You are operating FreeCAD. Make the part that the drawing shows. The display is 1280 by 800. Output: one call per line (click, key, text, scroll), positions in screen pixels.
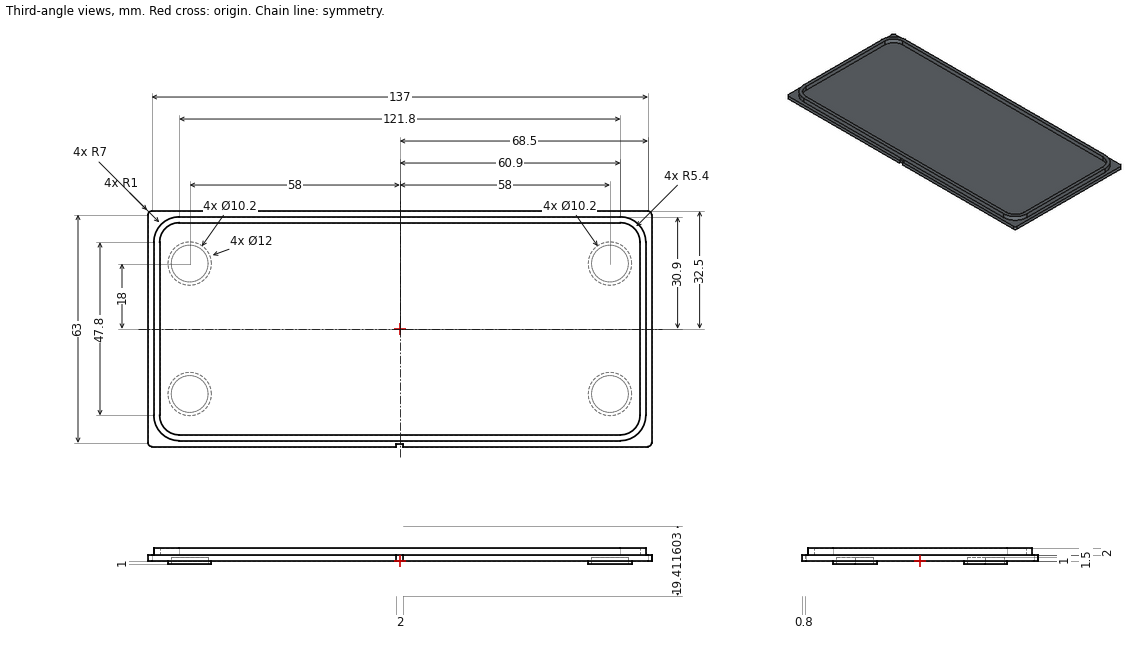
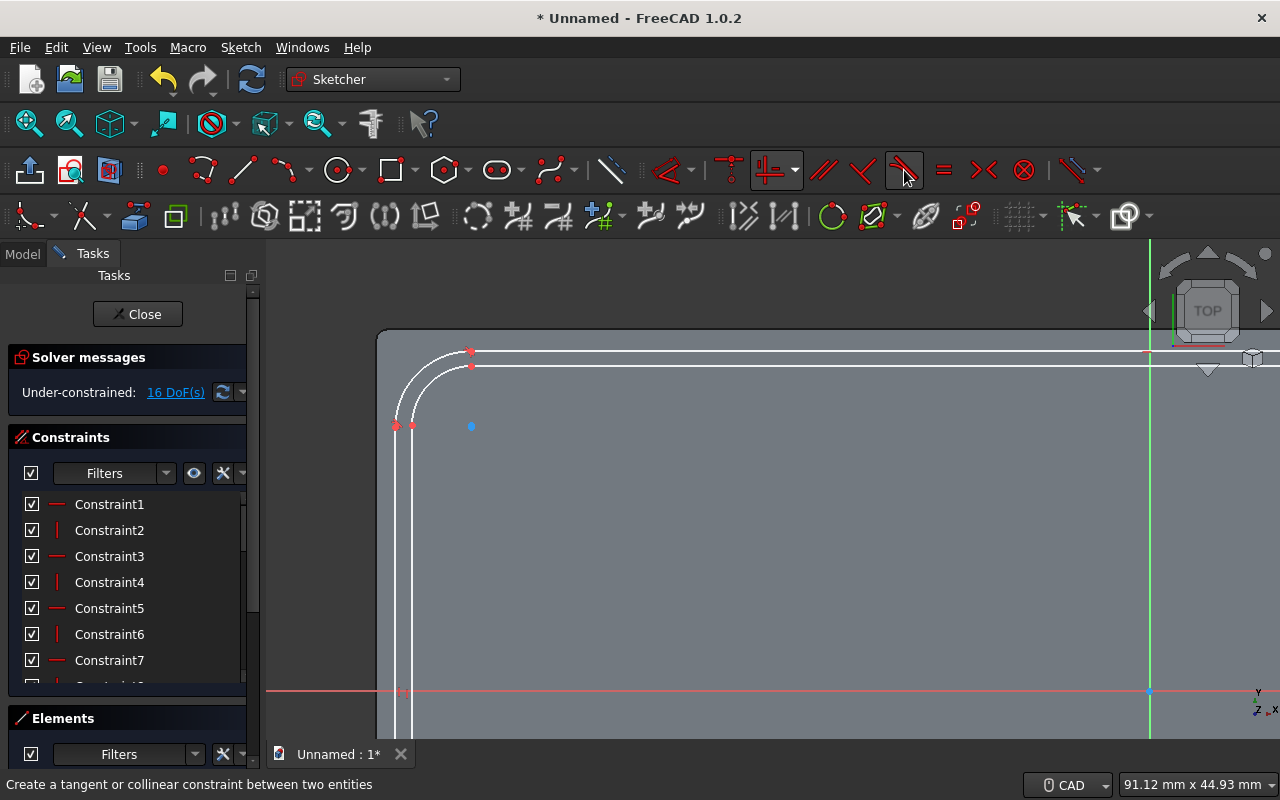
scroll(445, 371, down, 5)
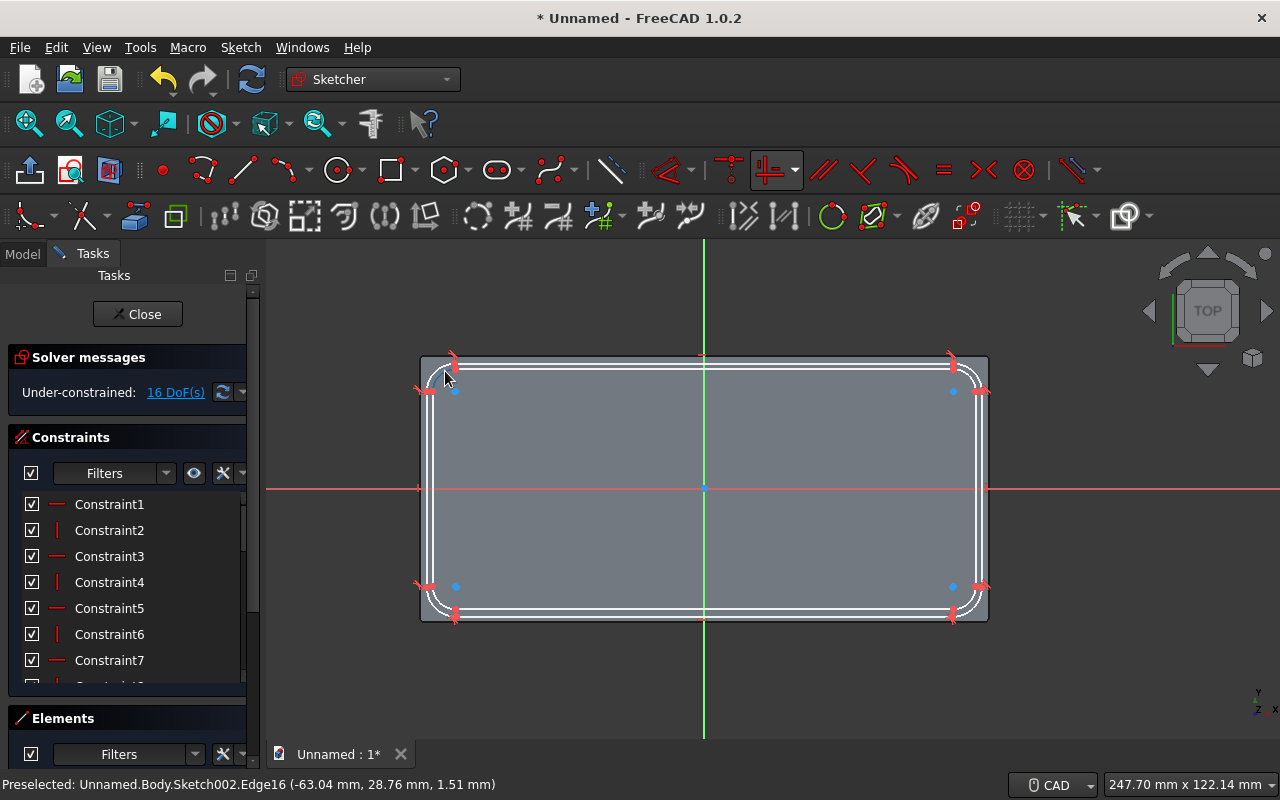
scroll(979, 379, up, 5)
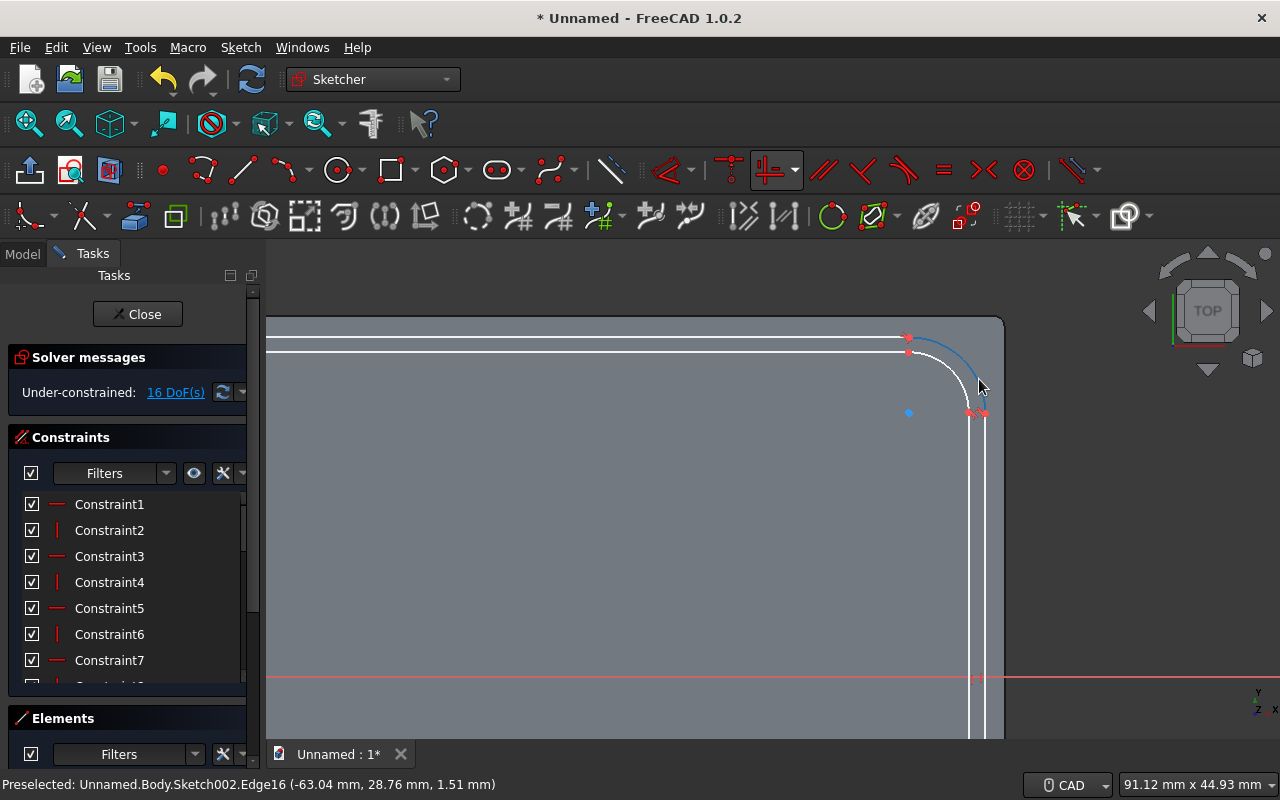
click(977, 379)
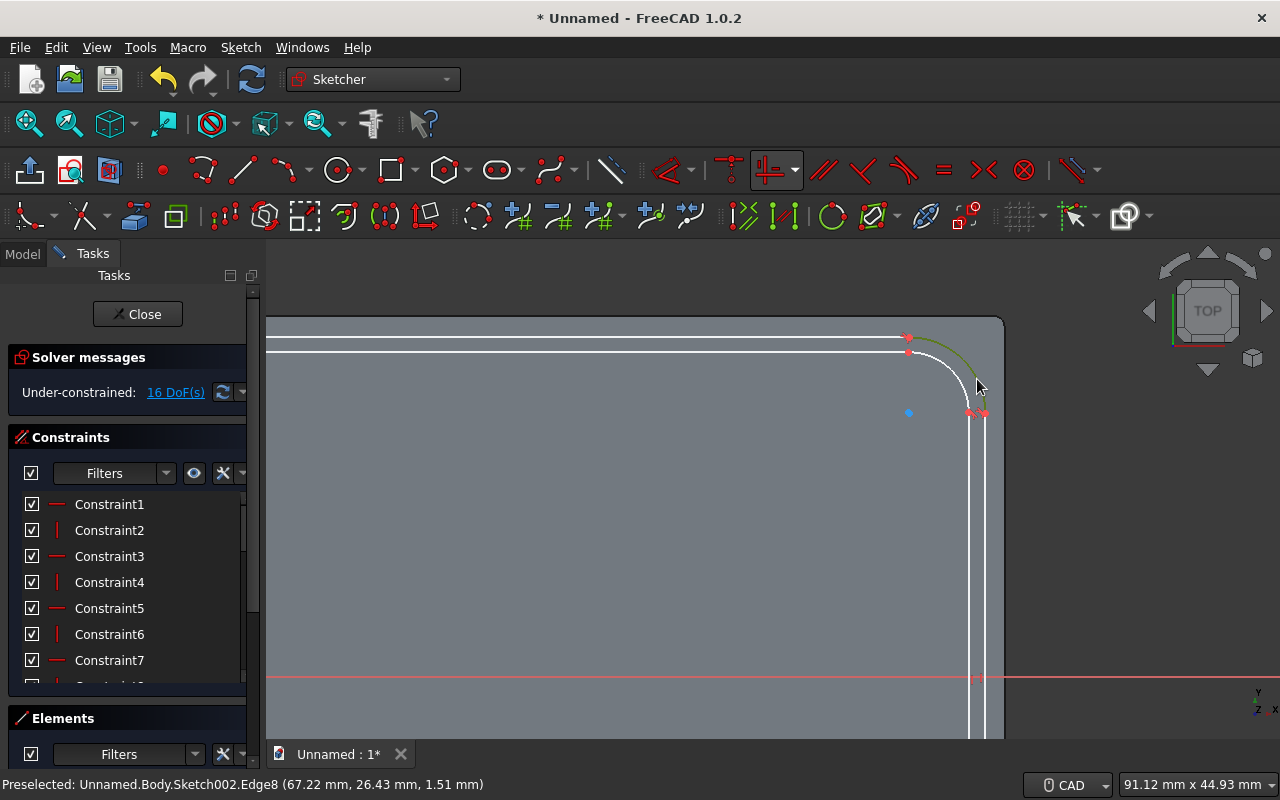
click(962, 385)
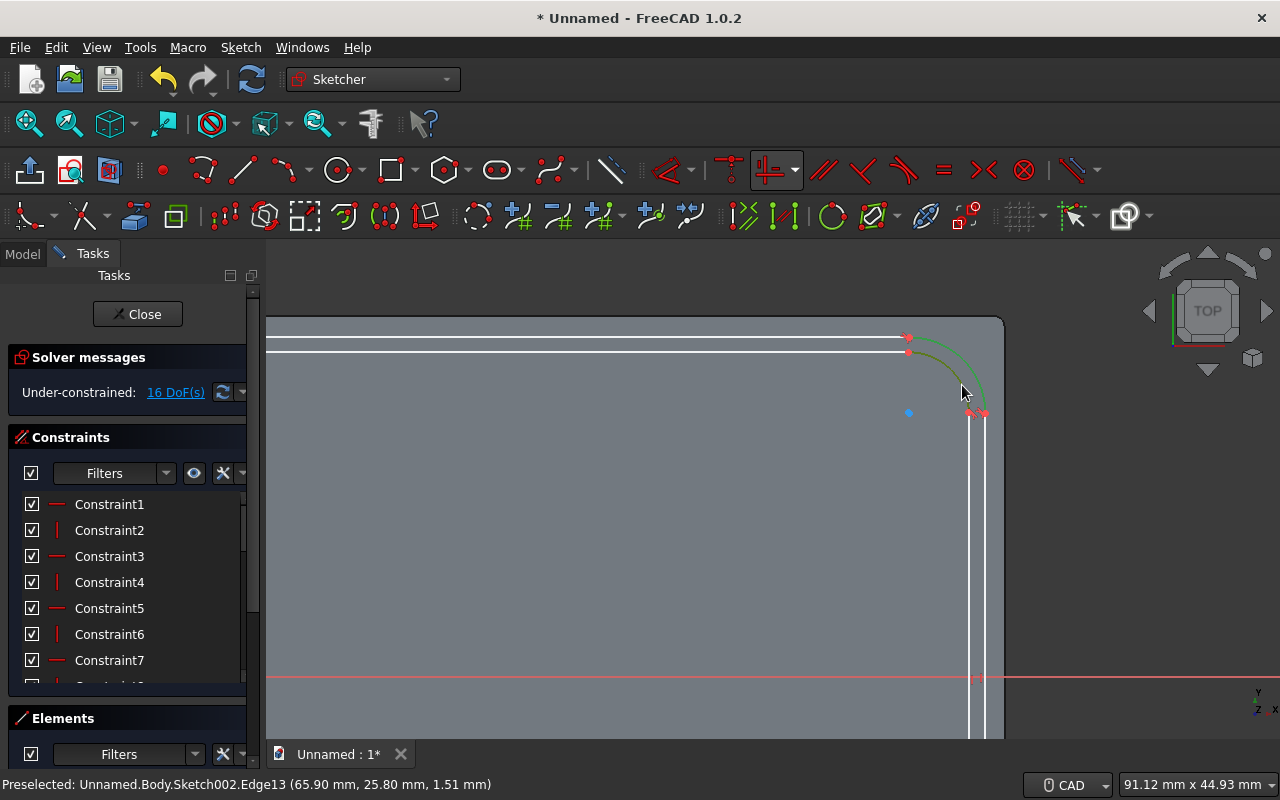
click(730, 170)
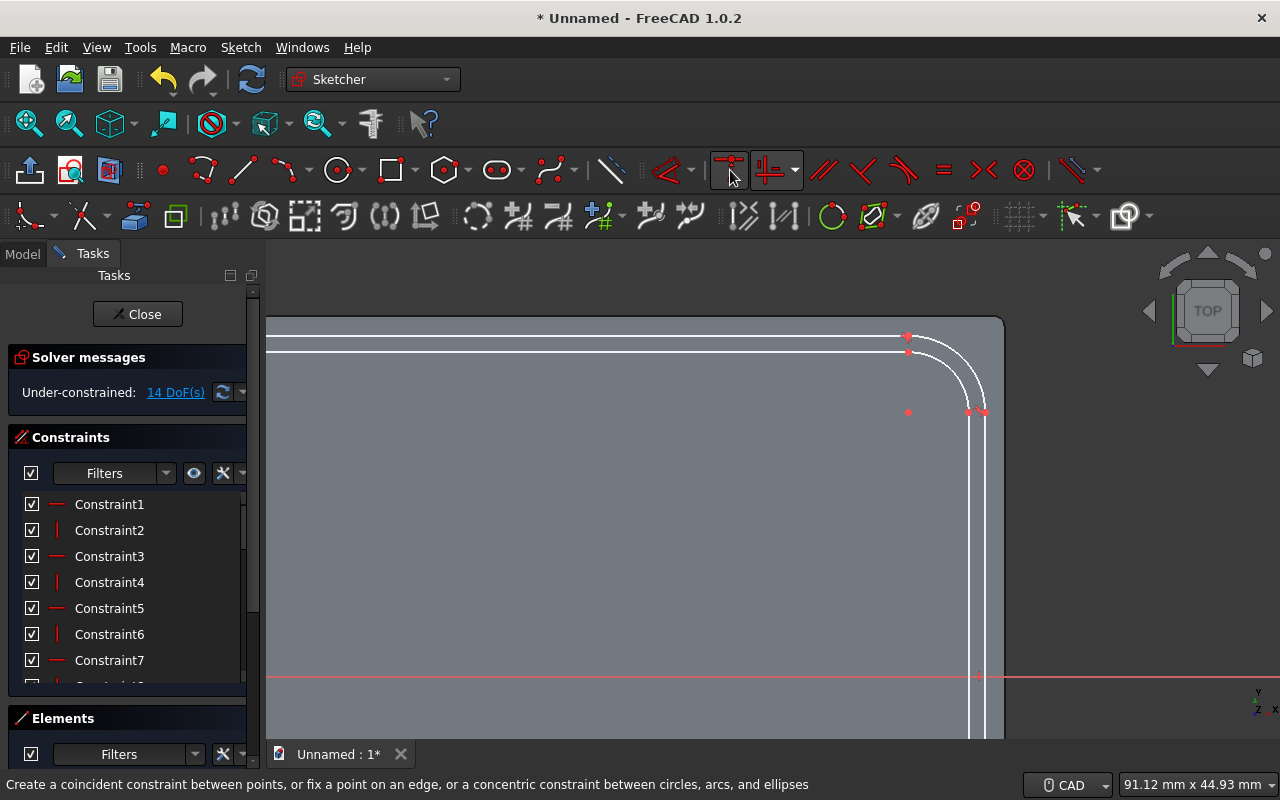
scroll(980, 379, down, 5)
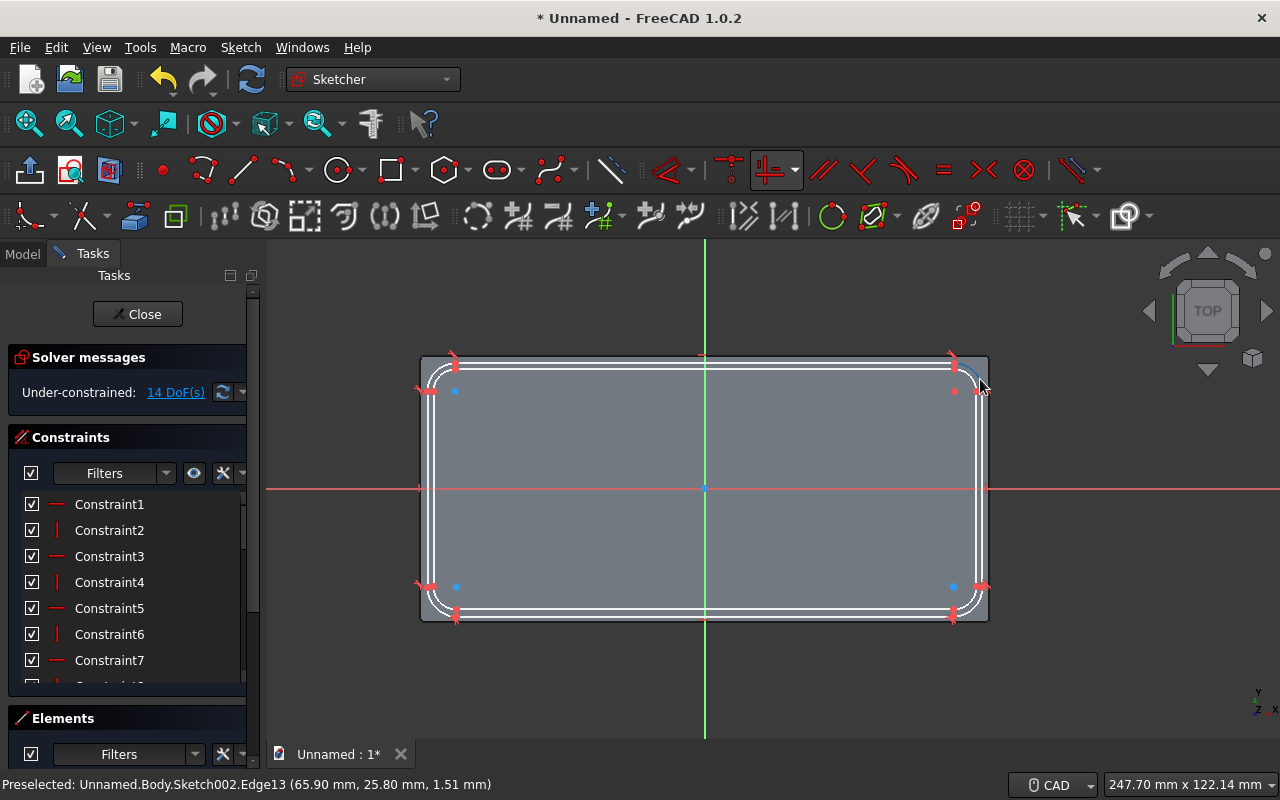
scroll(966, 614, up, 4)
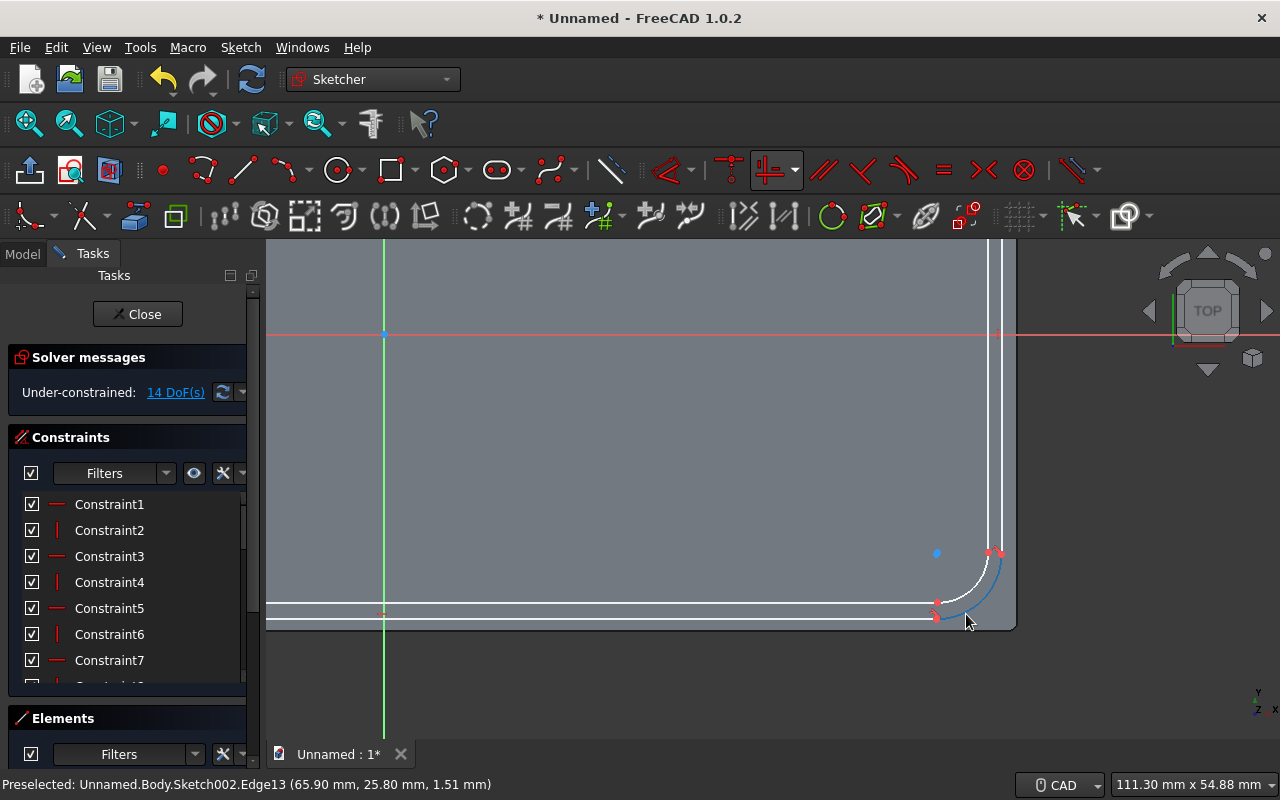
click(966, 612)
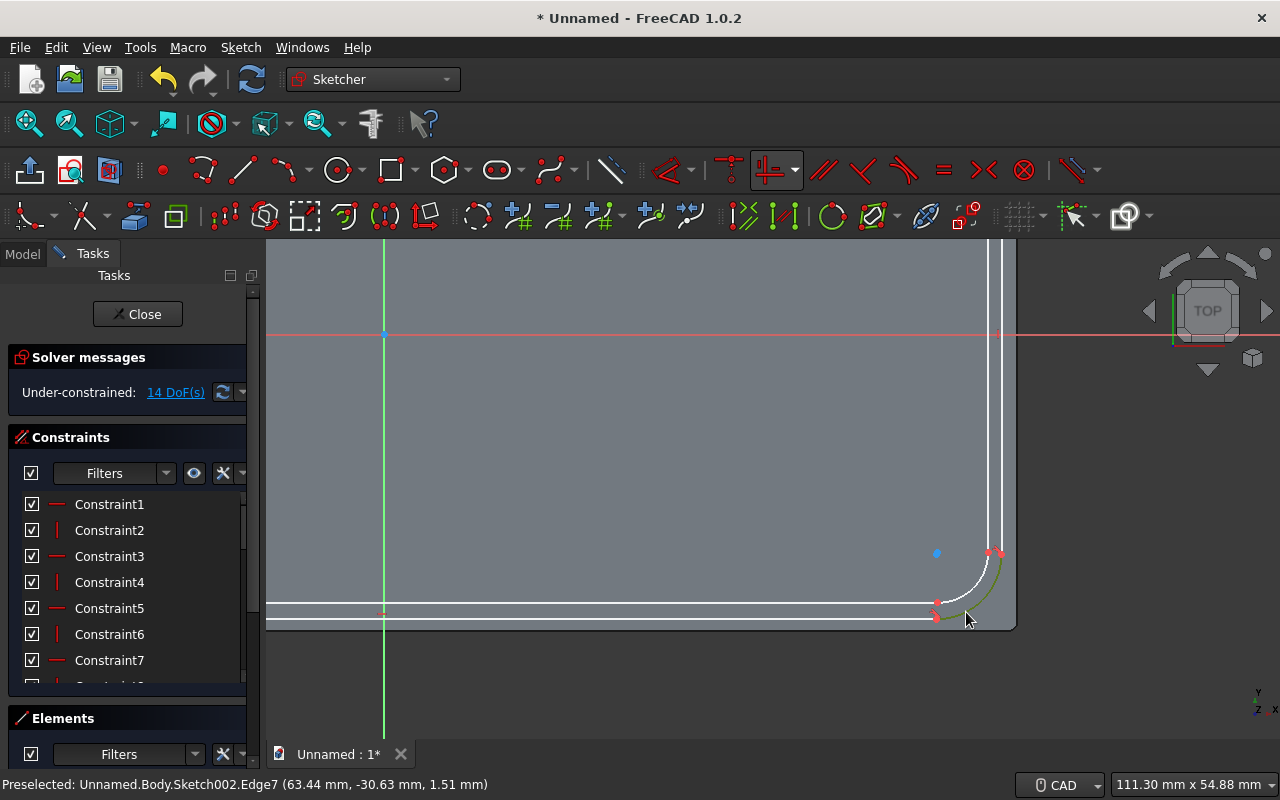
click(961, 597)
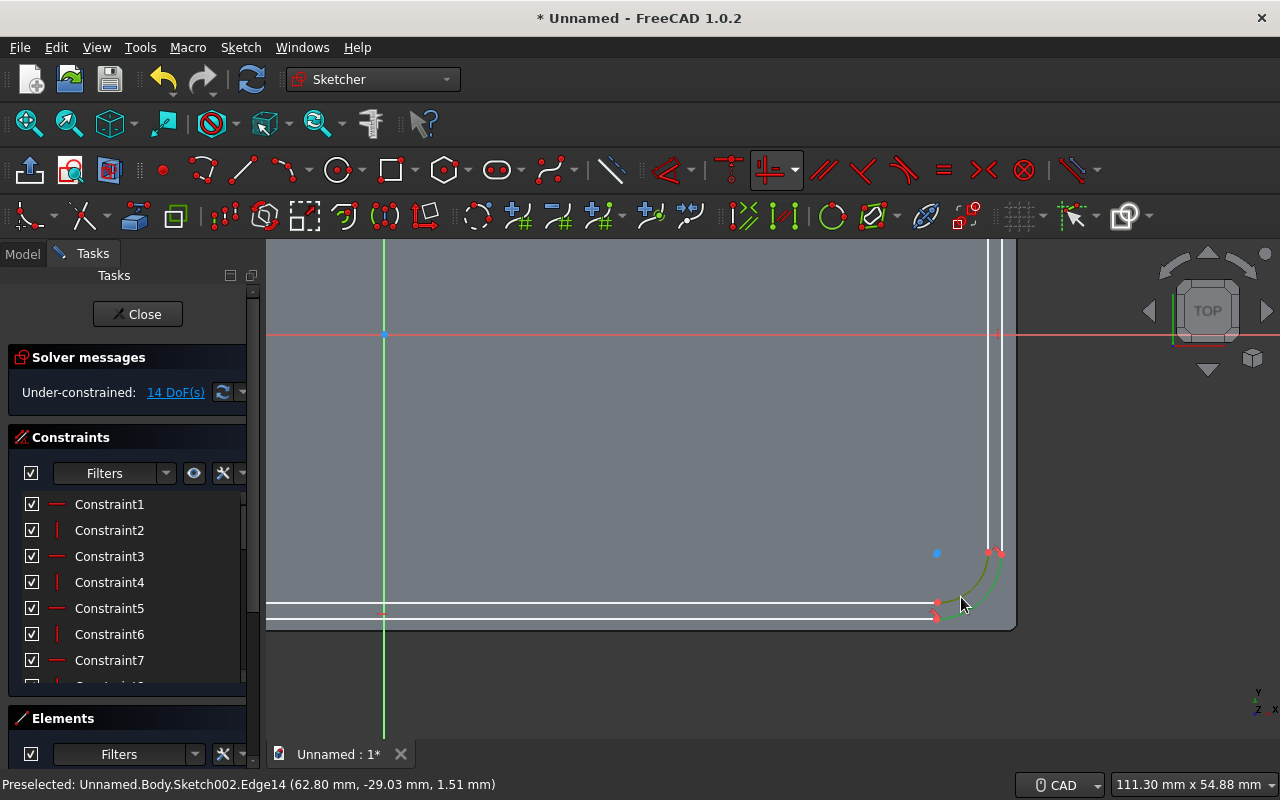
click(730, 170)